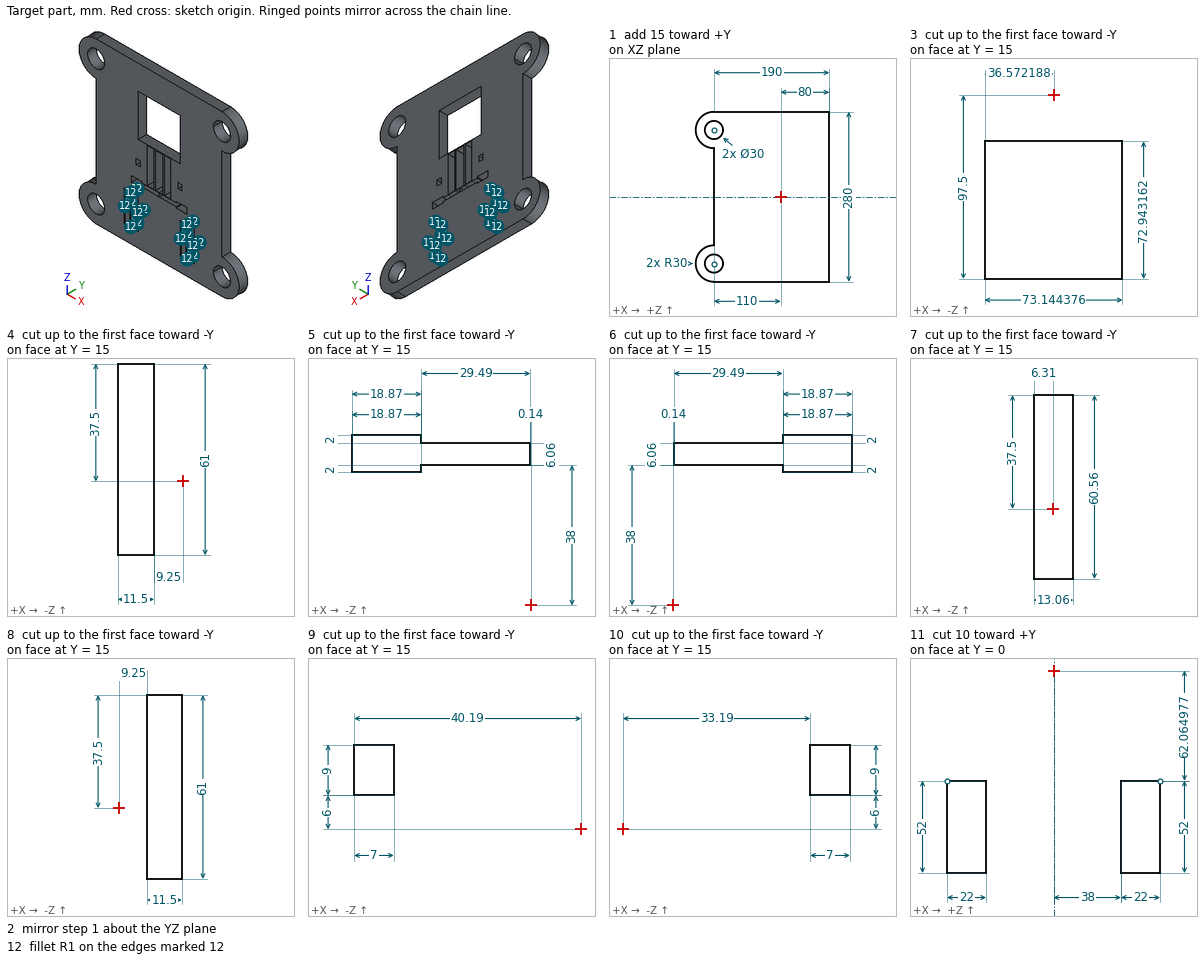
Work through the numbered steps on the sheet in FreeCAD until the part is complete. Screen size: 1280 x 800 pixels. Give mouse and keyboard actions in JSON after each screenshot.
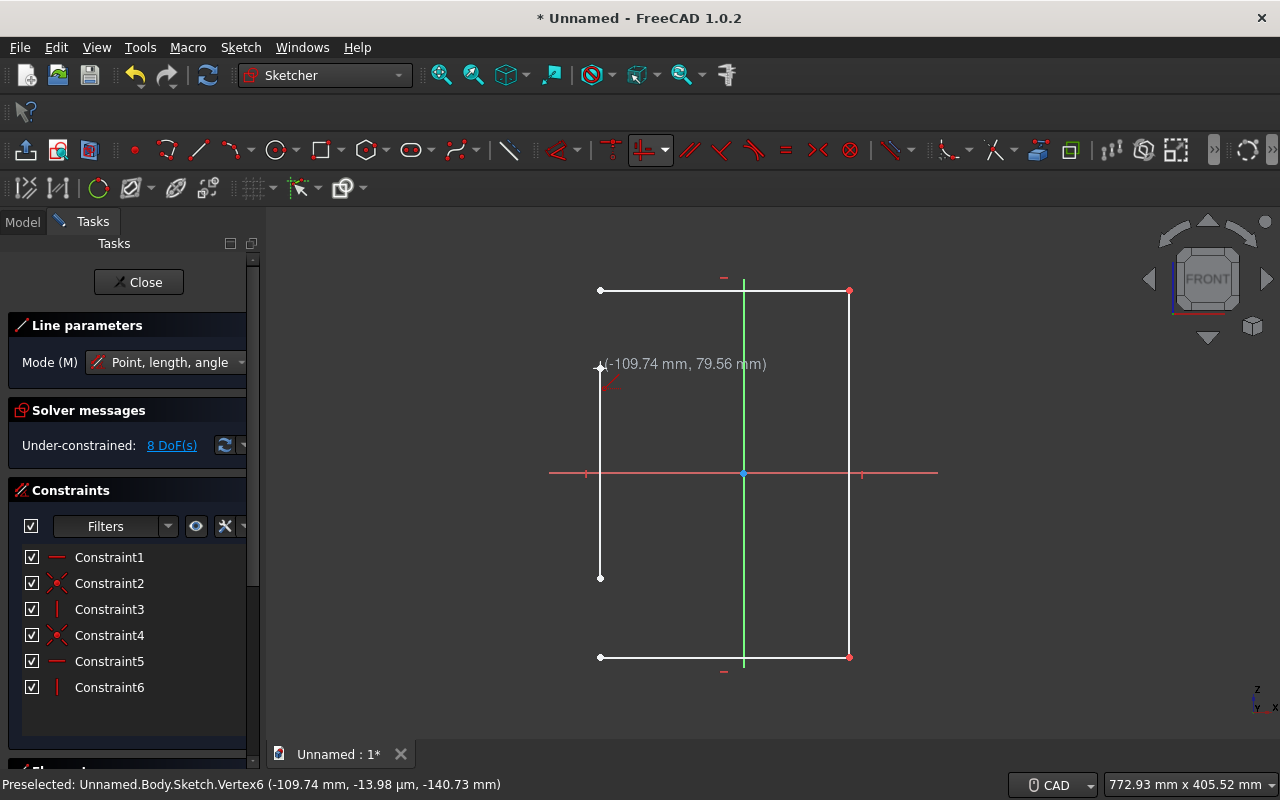
{"action": "key", "text": "g 3 a"}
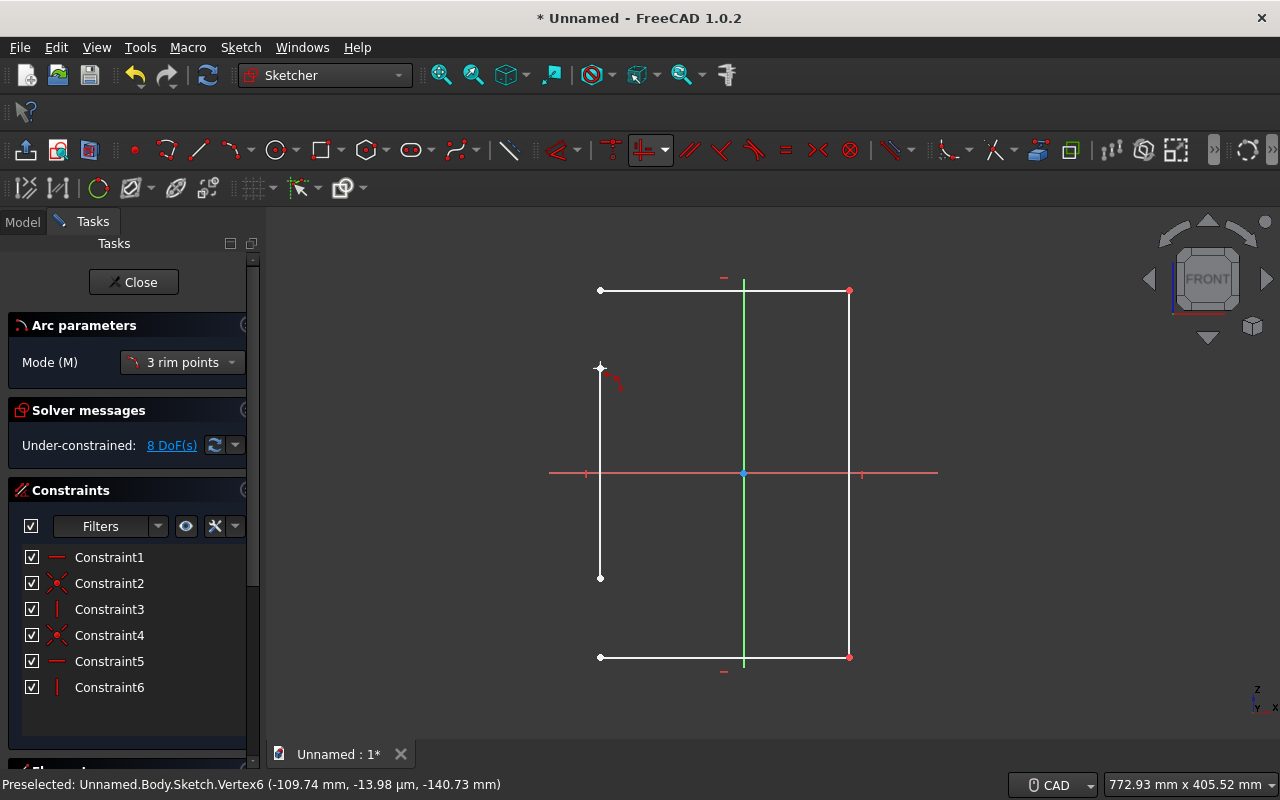
{"action": "left_click", "coordinate": [600, 658]}
{"action": "left_click", "coordinate": [600, 579]}
{"action": "left_click", "coordinate": [560, 618]}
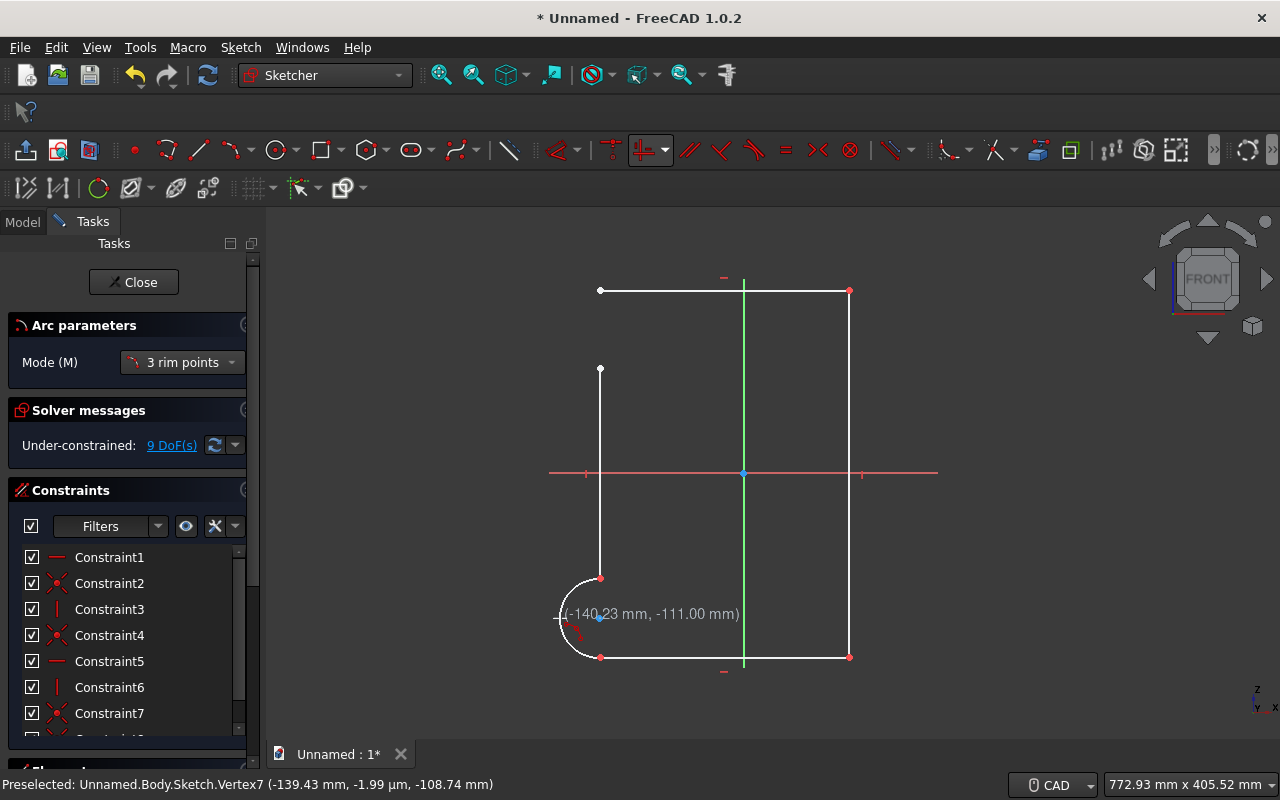
{"action": "left_click", "coordinate": [600, 369]}
{"action": "left_click", "coordinate": [600, 291]}
{"action": "left_click", "coordinate": [560, 329]}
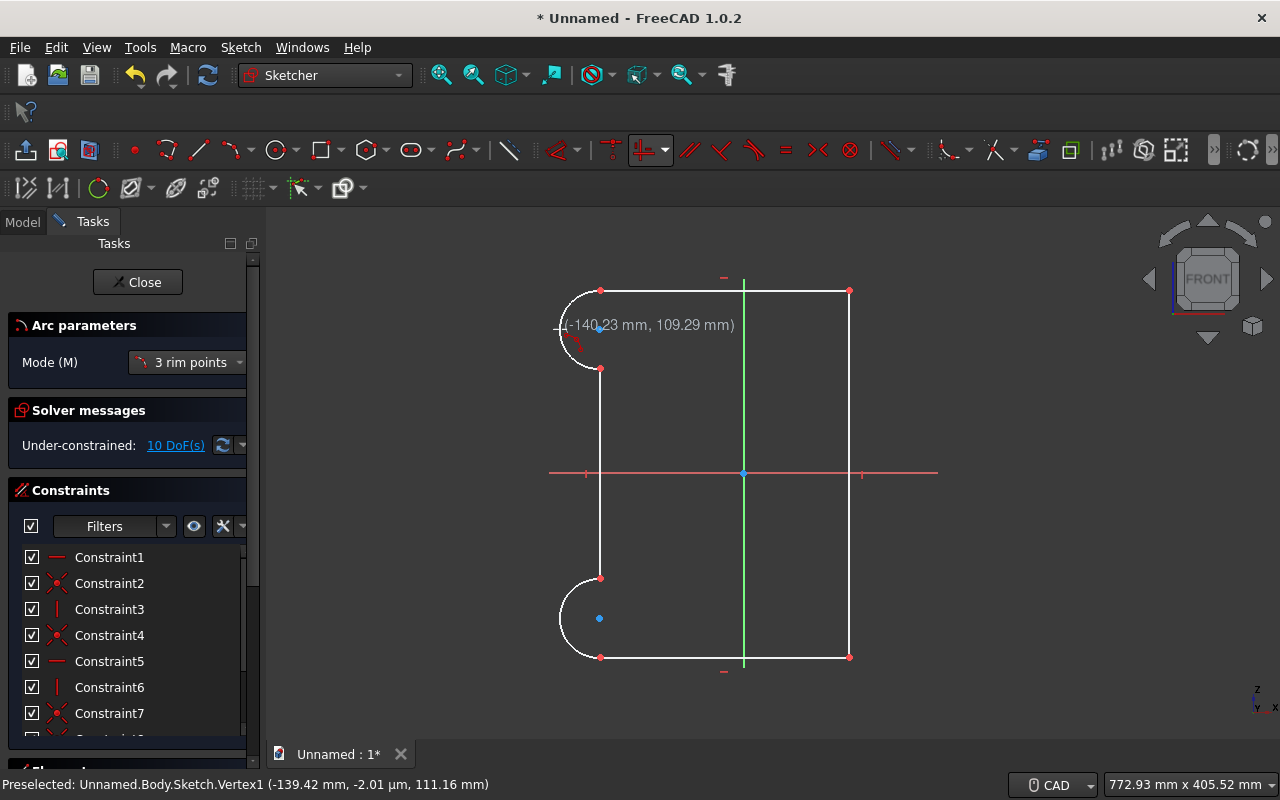
{"action": "left_click", "coordinate": [276, 150]}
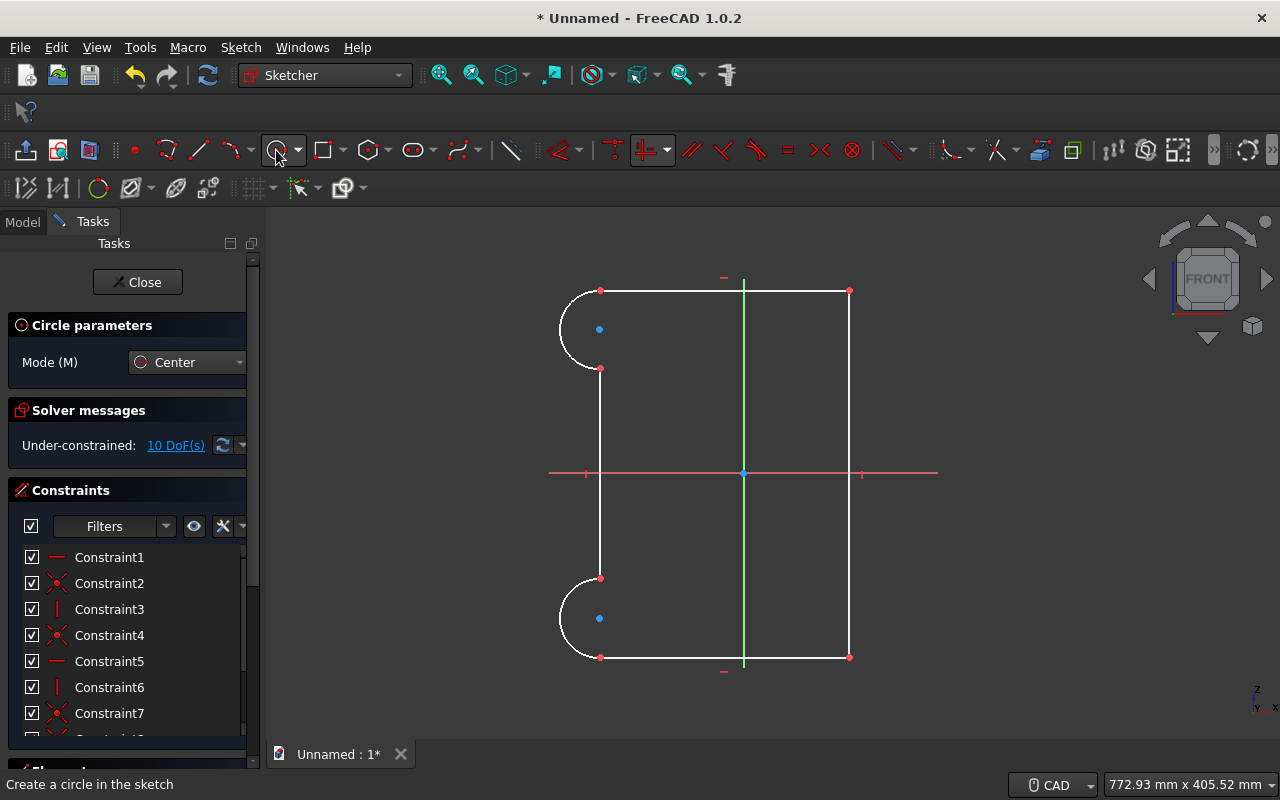
{"action": "left_click", "coordinate": [600, 329]}
{"action": "mouse_move", "coordinate": [614, 315]}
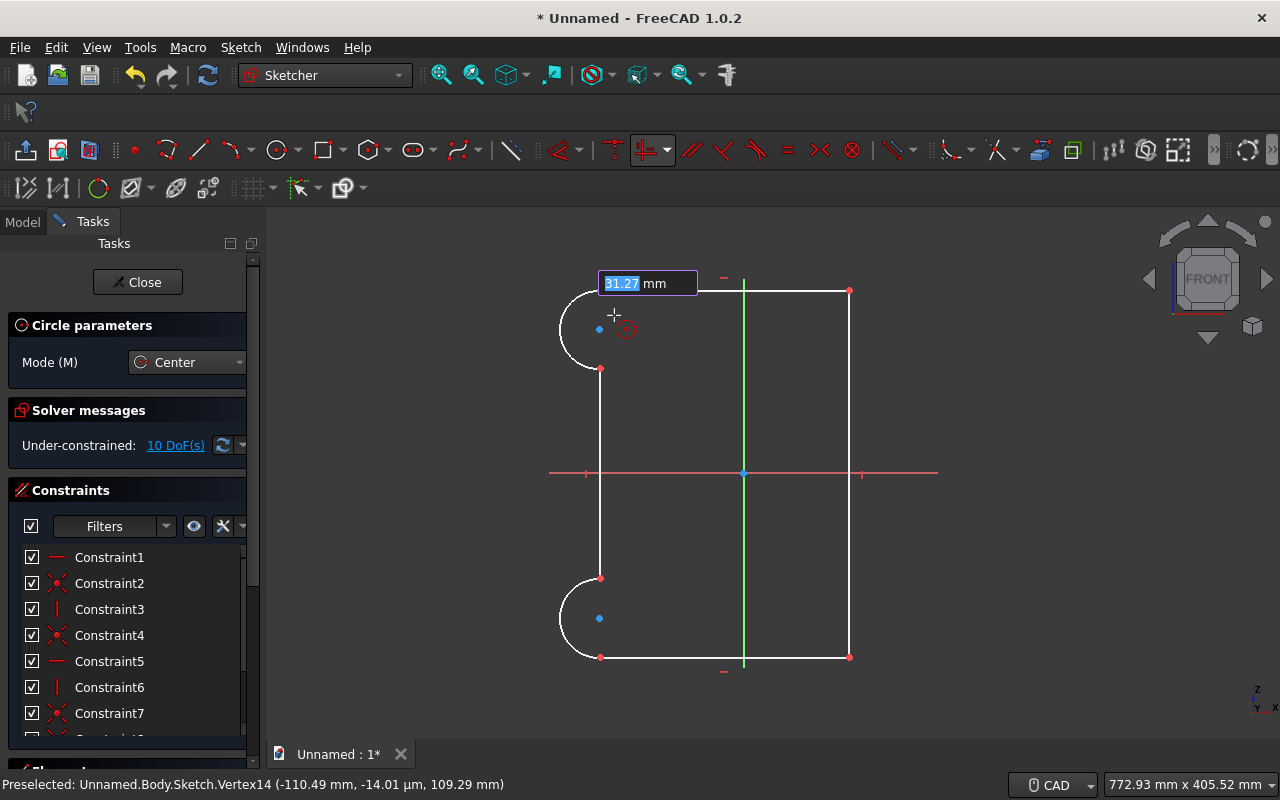
{"action": "type", "text": "30"}
{"action": "key", "text": "Return"}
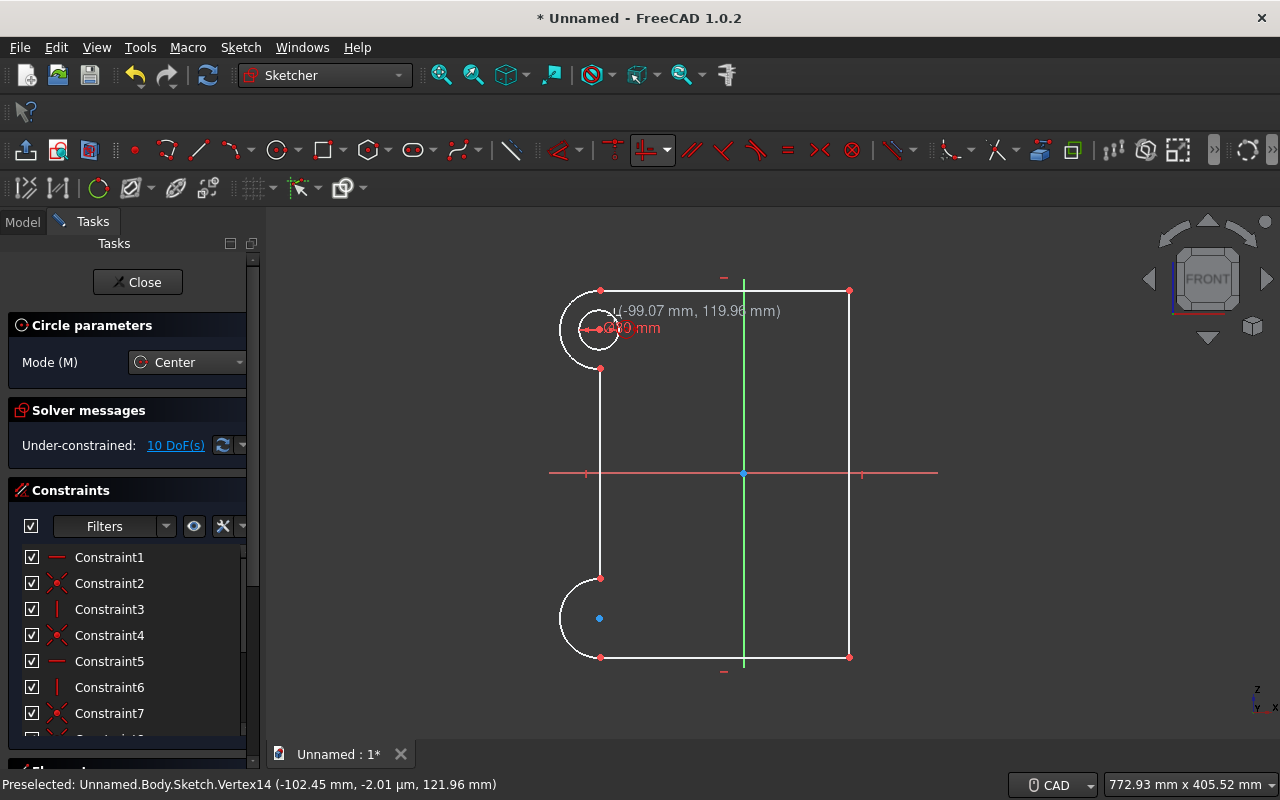
{"action": "left_click", "coordinate": [600, 618]}
{"action": "mouse_move", "coordinate": [614, 604]}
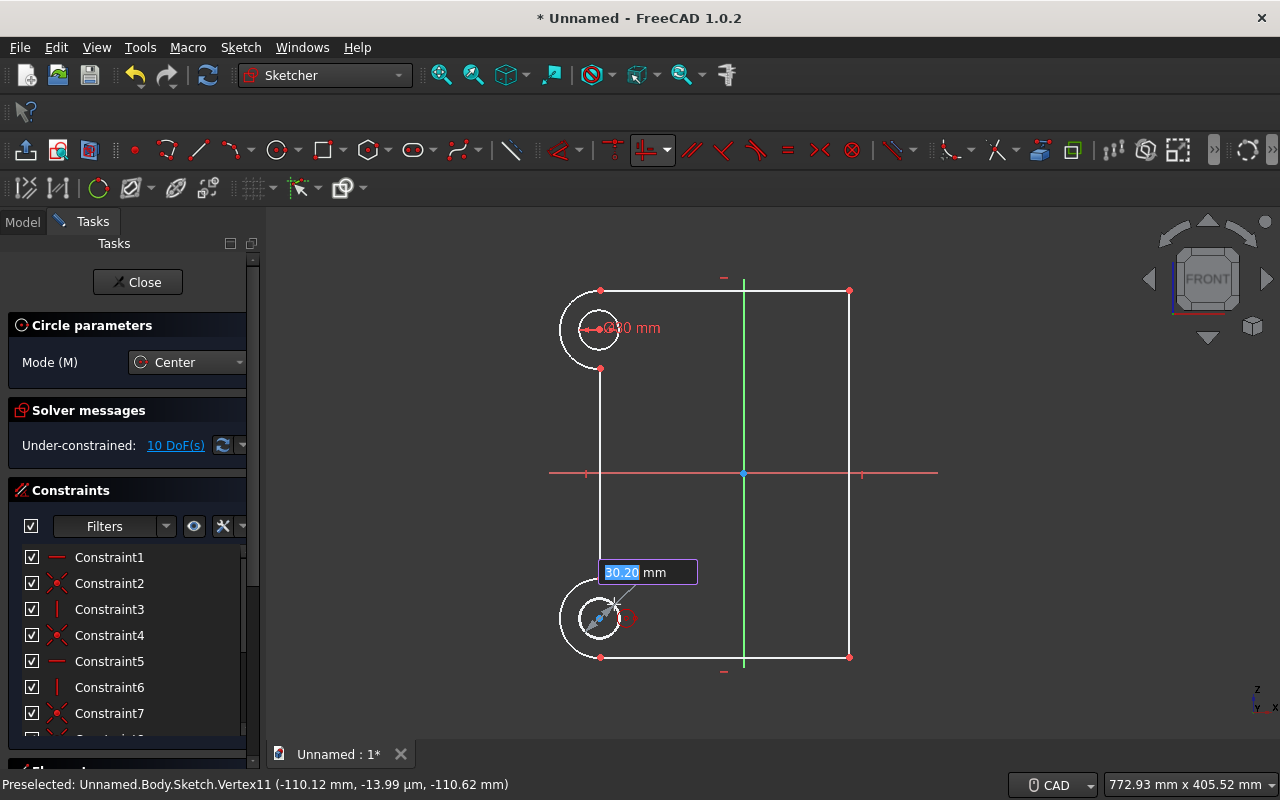
{"action": "type", "text": "30"}
{"action": "key", "text": "Return"}
{"action": "key", "text": "Escape"}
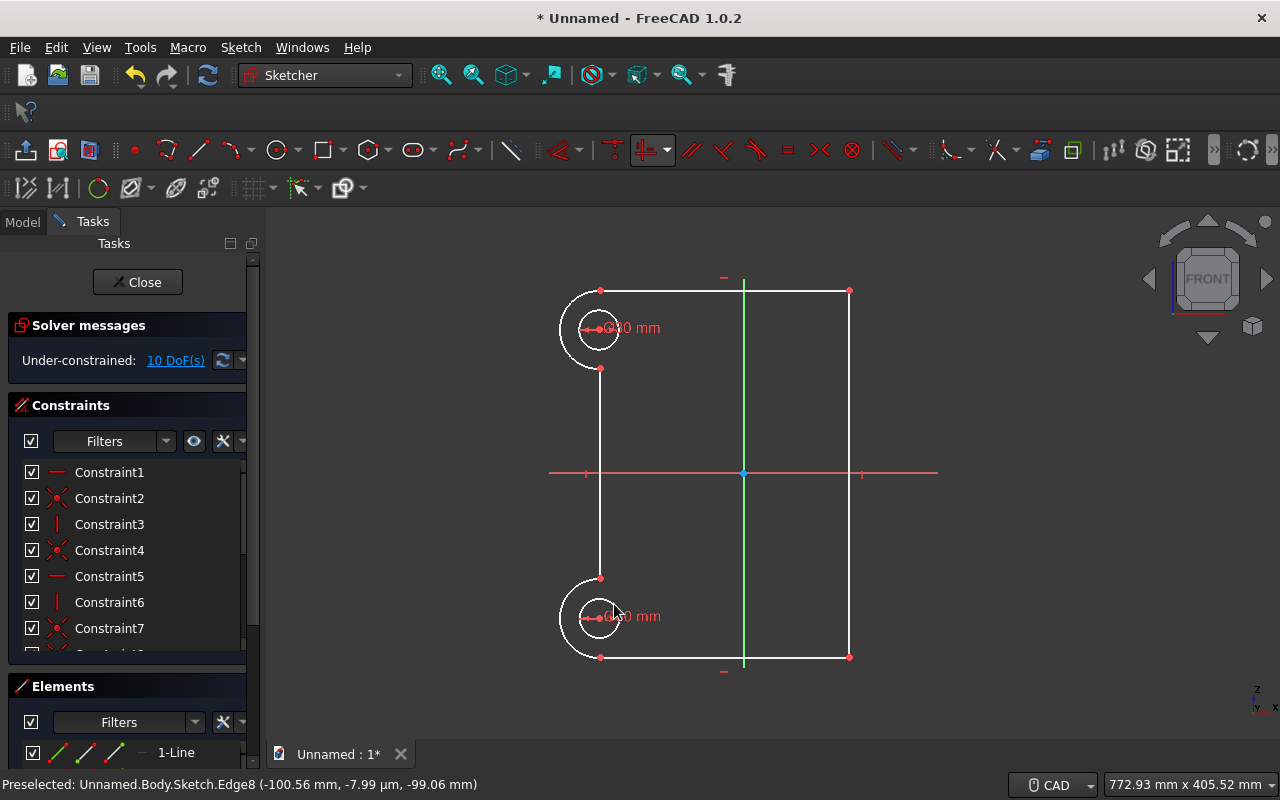
{"action": "left_click", "coordinate": [675, 291]}